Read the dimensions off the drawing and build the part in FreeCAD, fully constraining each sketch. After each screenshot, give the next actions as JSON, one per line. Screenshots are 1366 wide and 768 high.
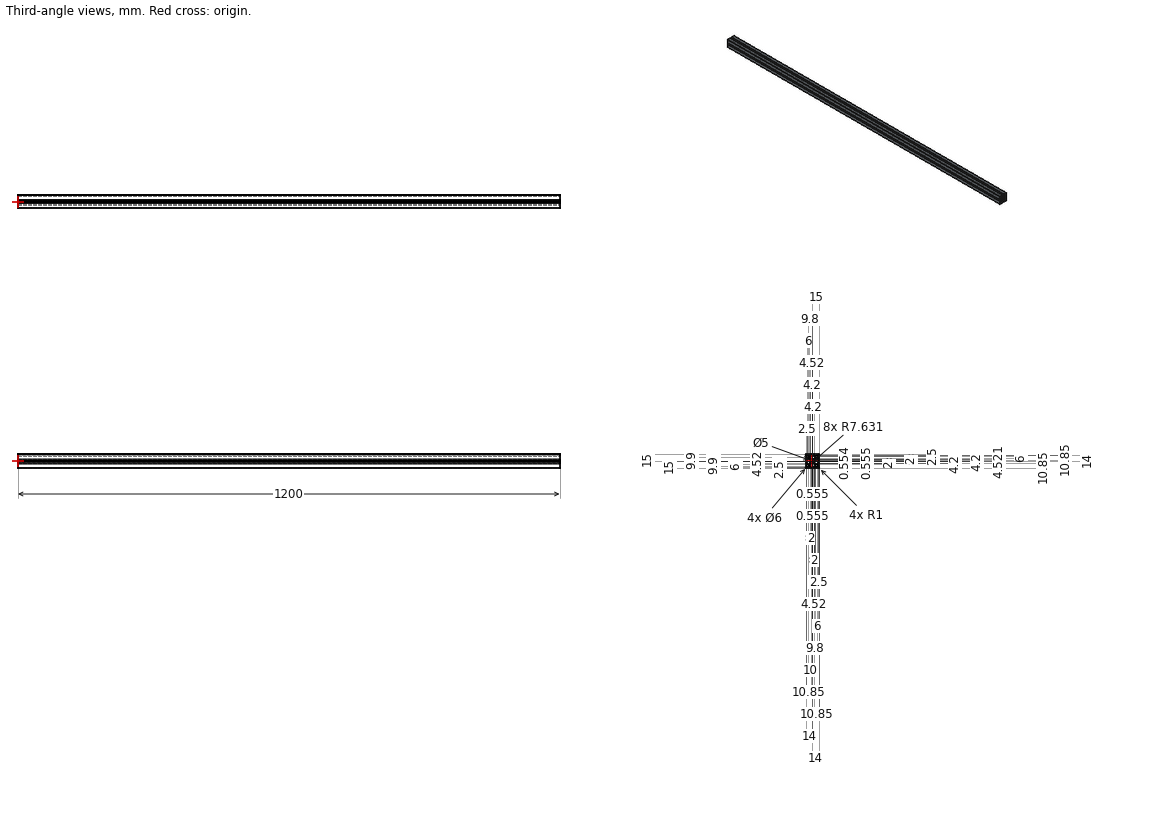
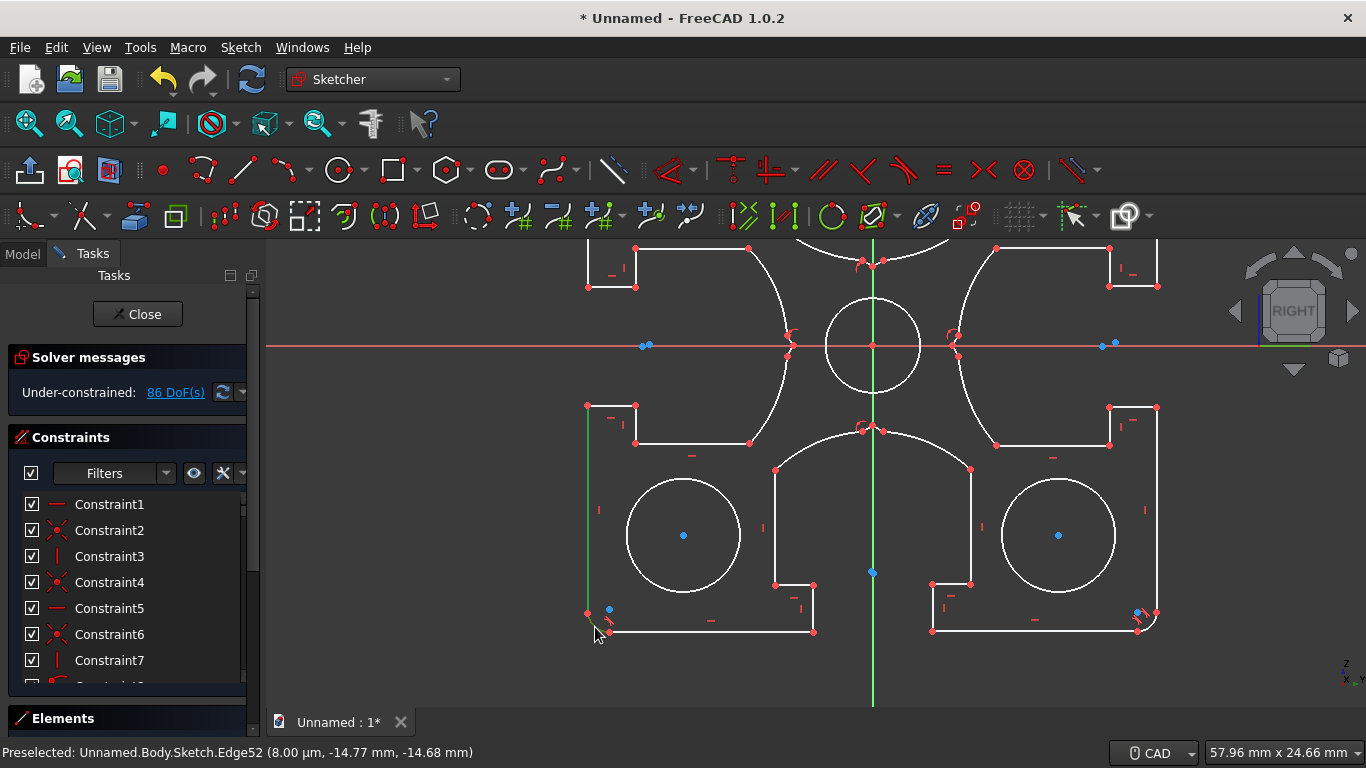
{"action": "left_click", "coordinate": [904, 170]}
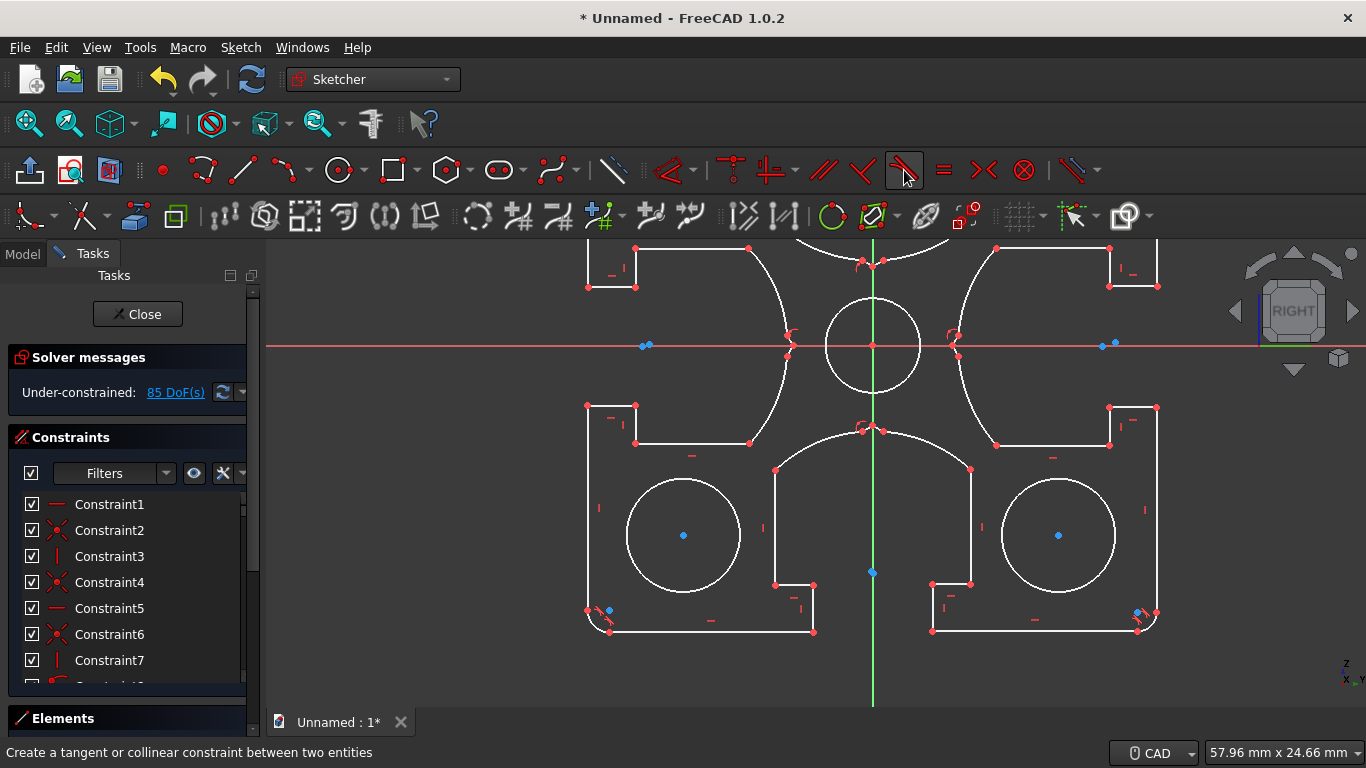
{"action": "left_click", "coordinate": [834, 437]}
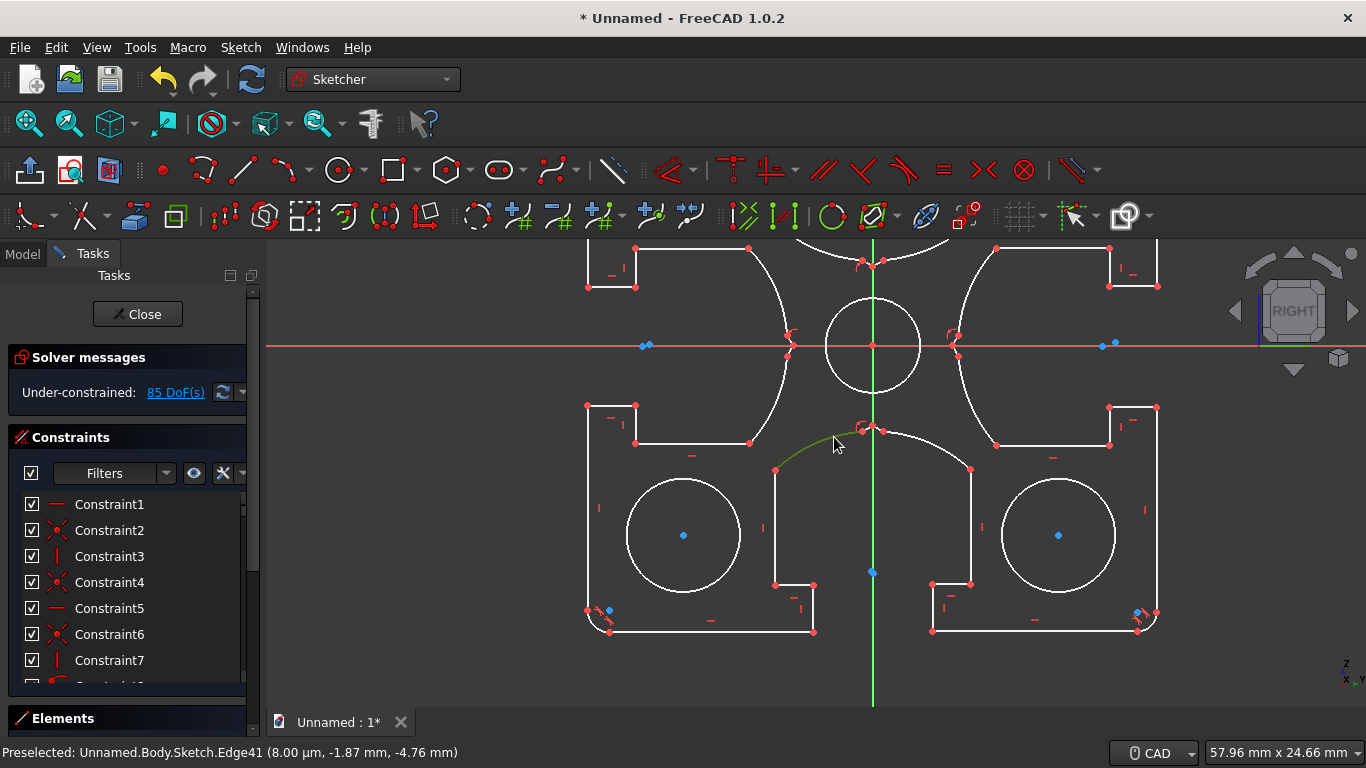
{"action": "left_click", "coordinate": [947, 452]}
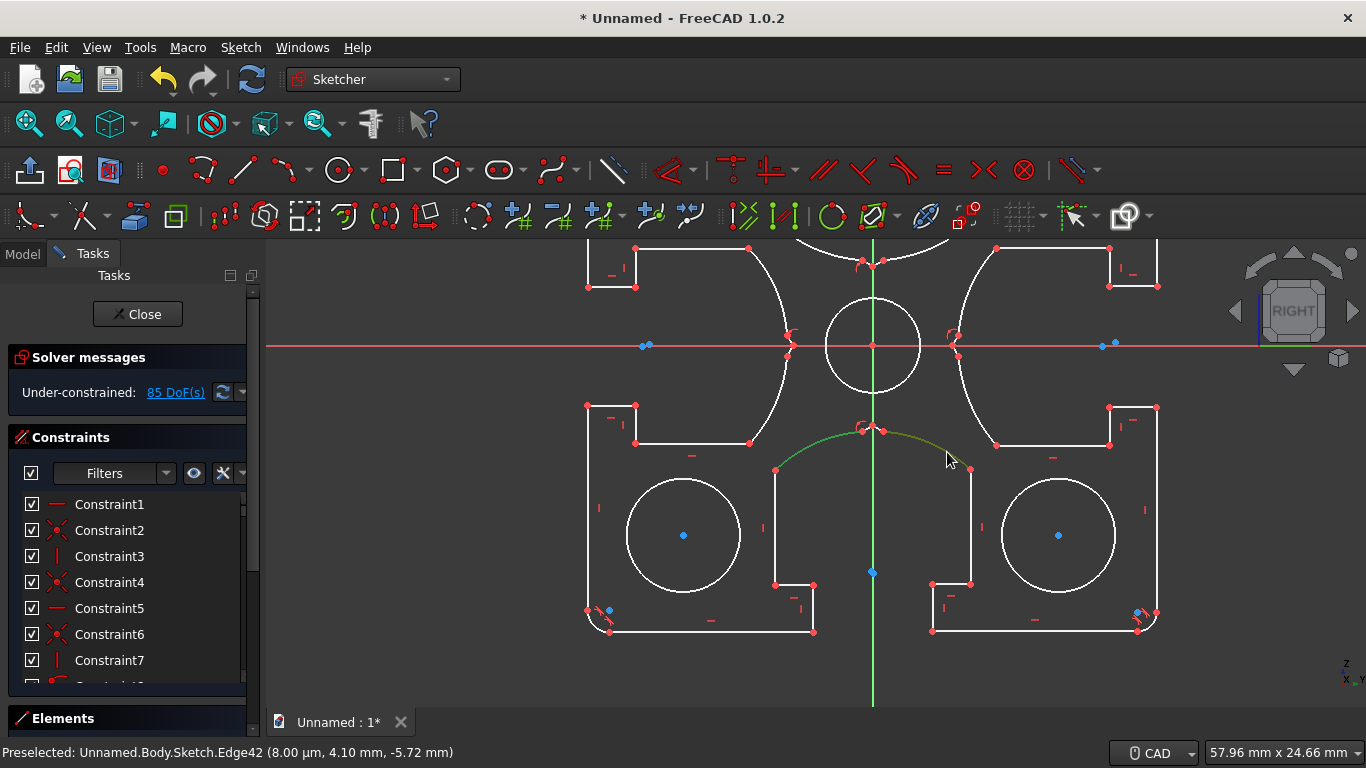
{"action": "left_click", "coordinate": [964, 385]}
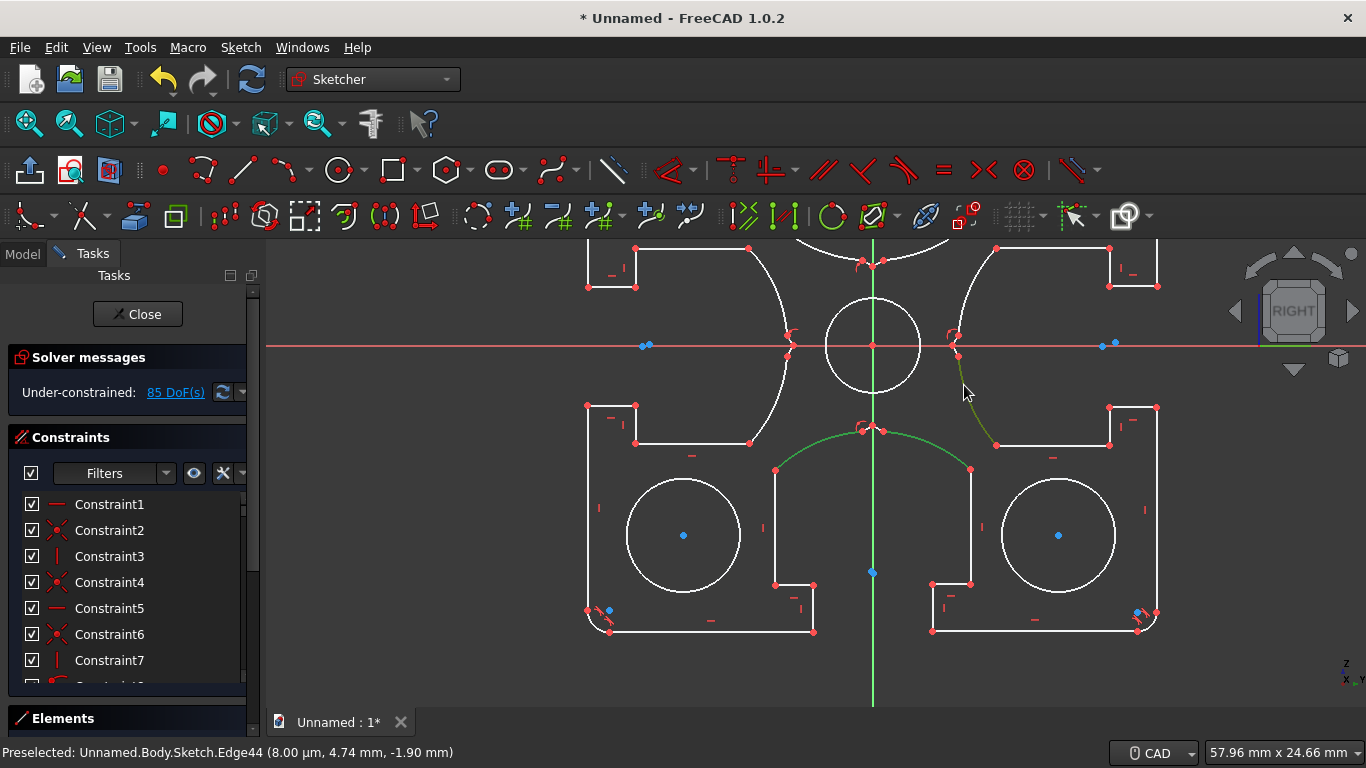
{"action": "left_click", "coordinate": [979, 271]}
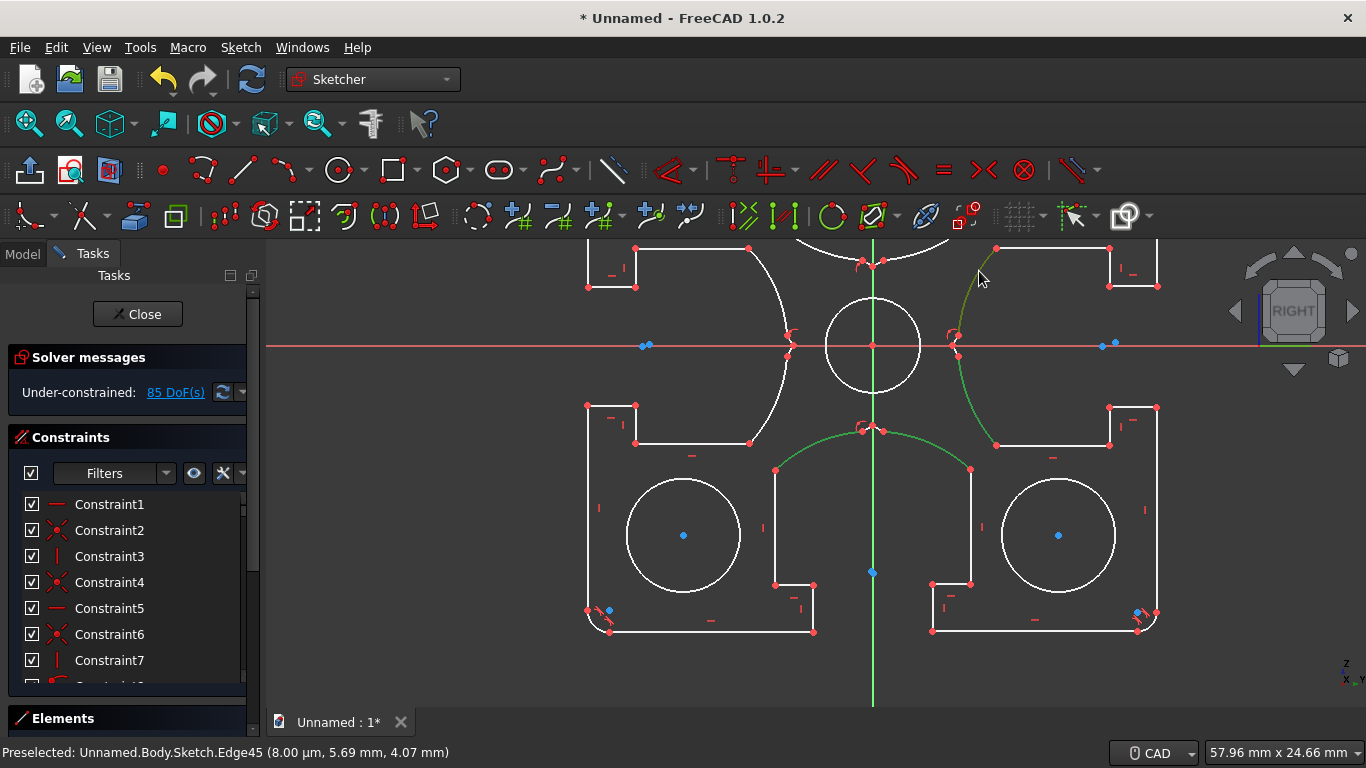
{"action": "scroll", "coordinate": [595, 628], "scroll_direction": "down", "scroll_amount": 3}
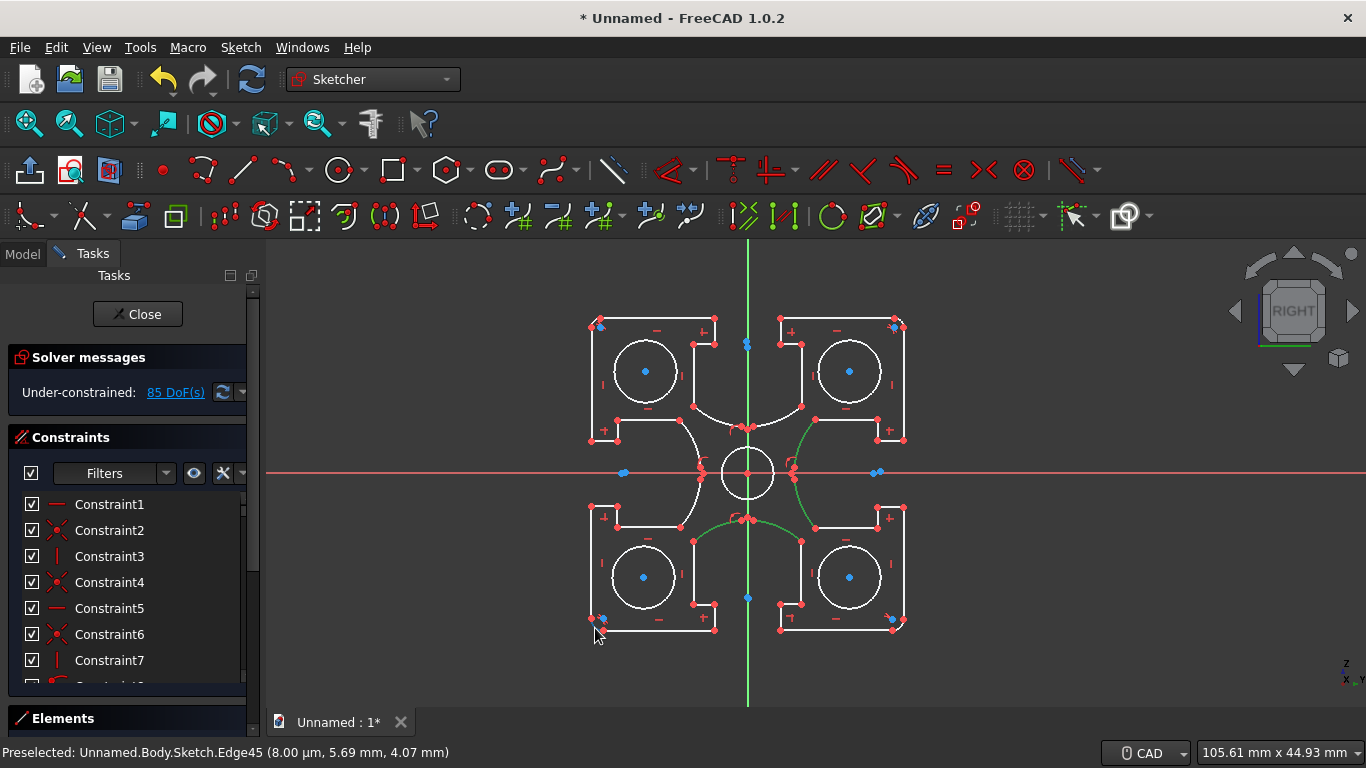
{"action": "left_click", "coordinate": [769, 424]}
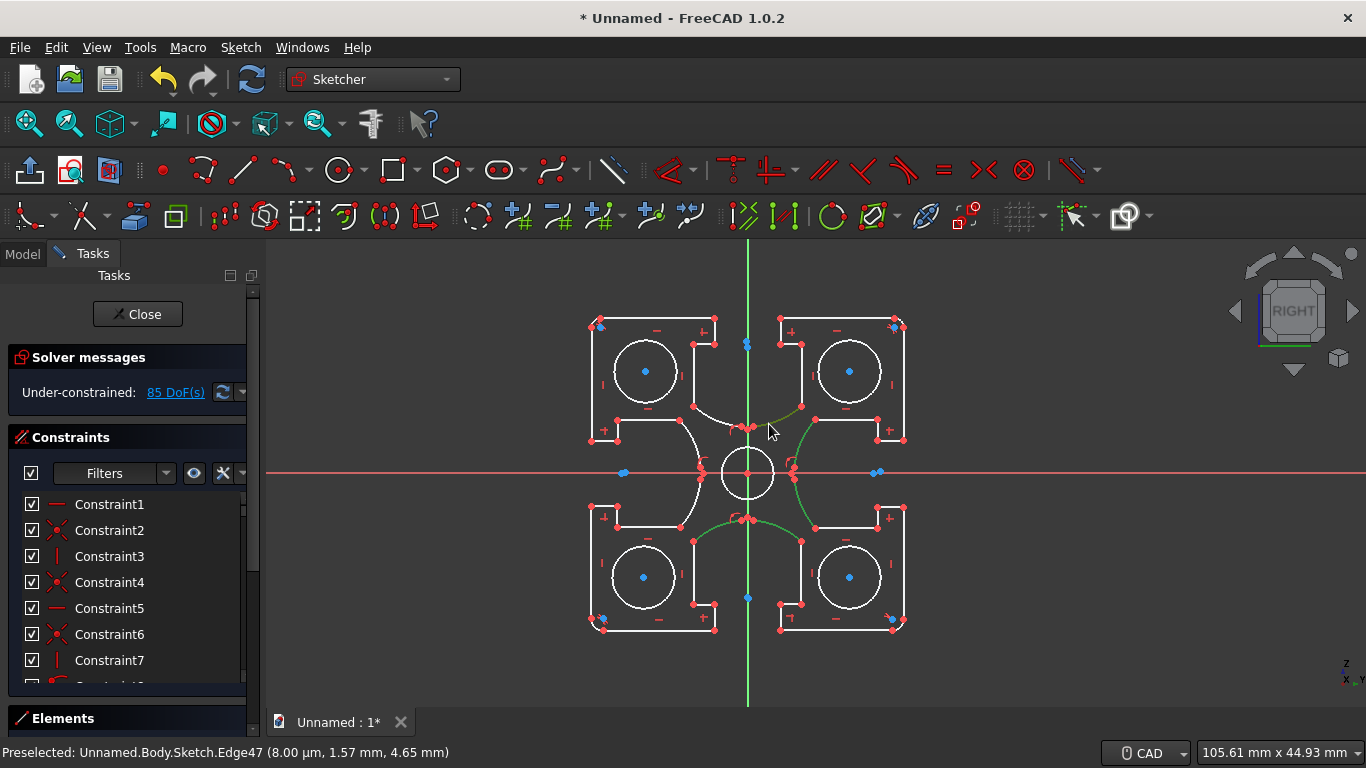
{"action": "left_click", "coordinate": [707, 416]}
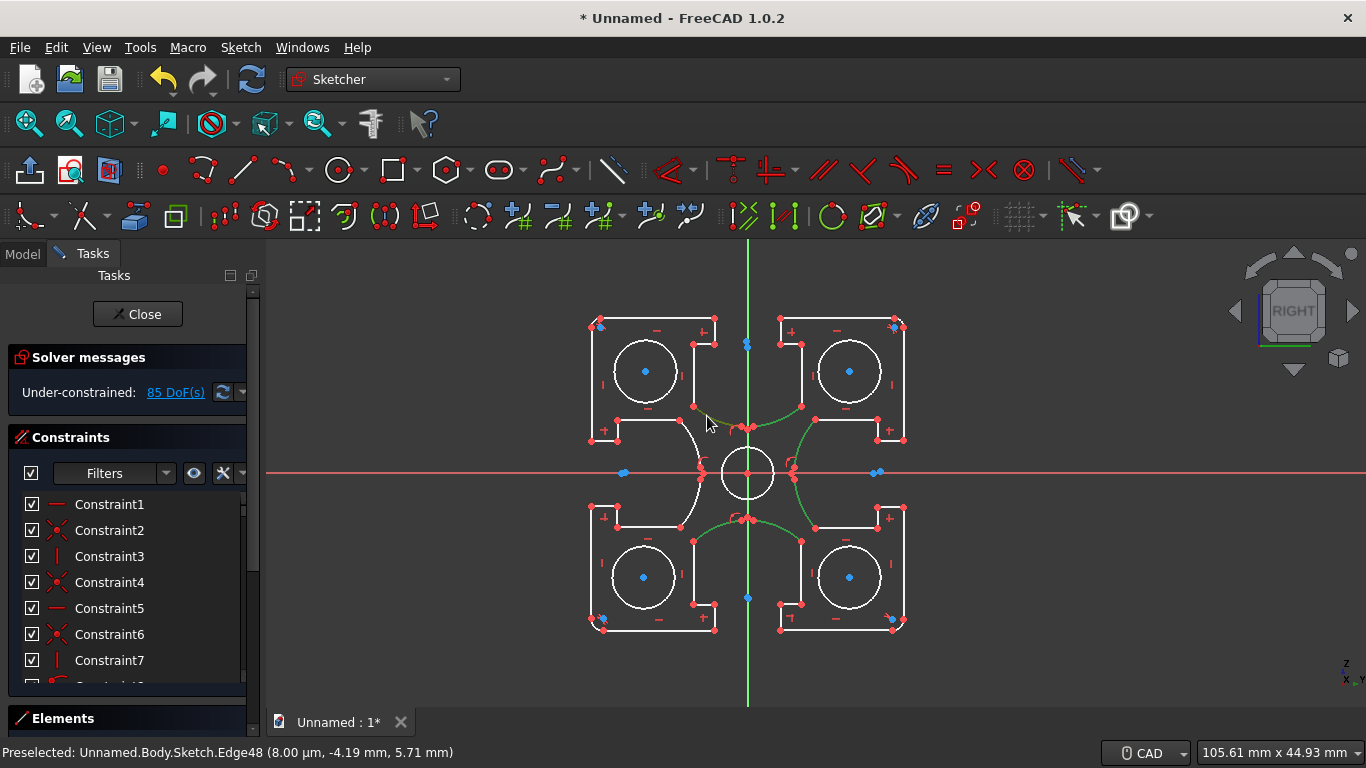
{"action": "left_click", "coordinate": [698, 452]}